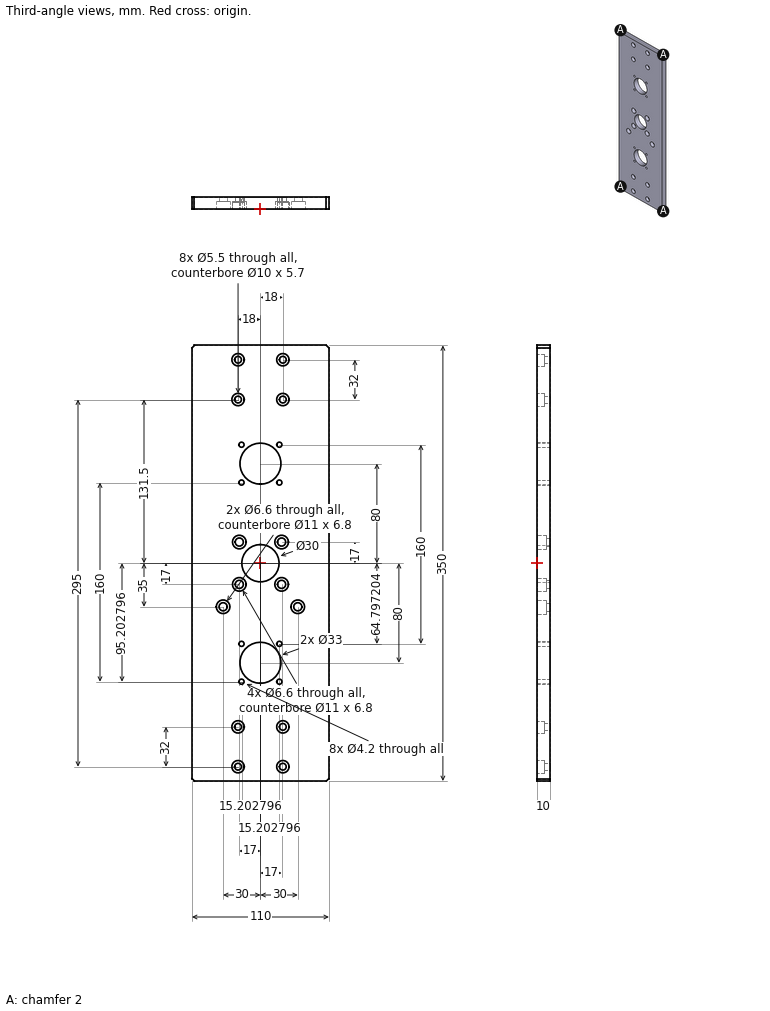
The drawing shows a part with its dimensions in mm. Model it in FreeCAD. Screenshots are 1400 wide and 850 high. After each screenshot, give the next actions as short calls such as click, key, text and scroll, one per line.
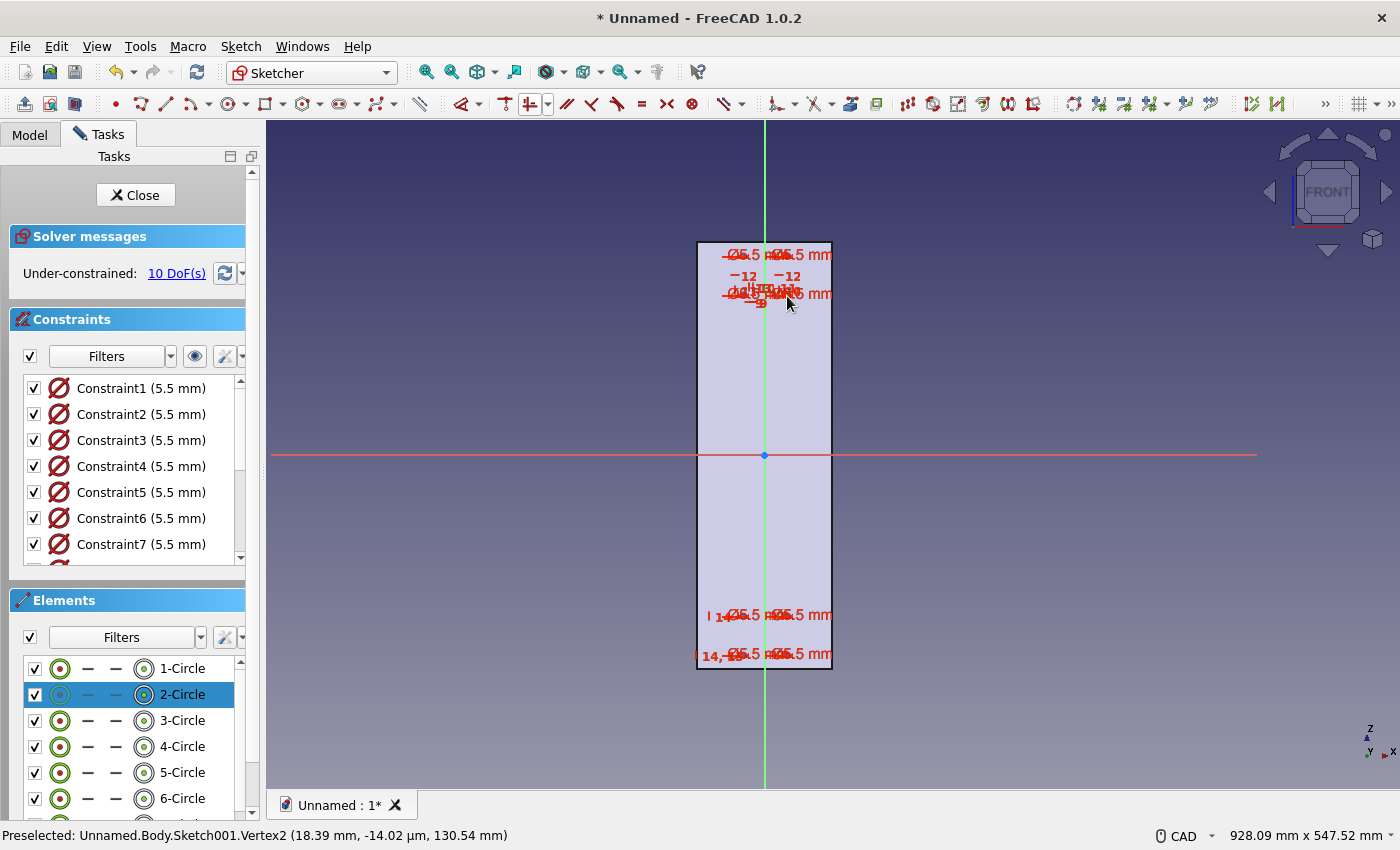
click(787, 656)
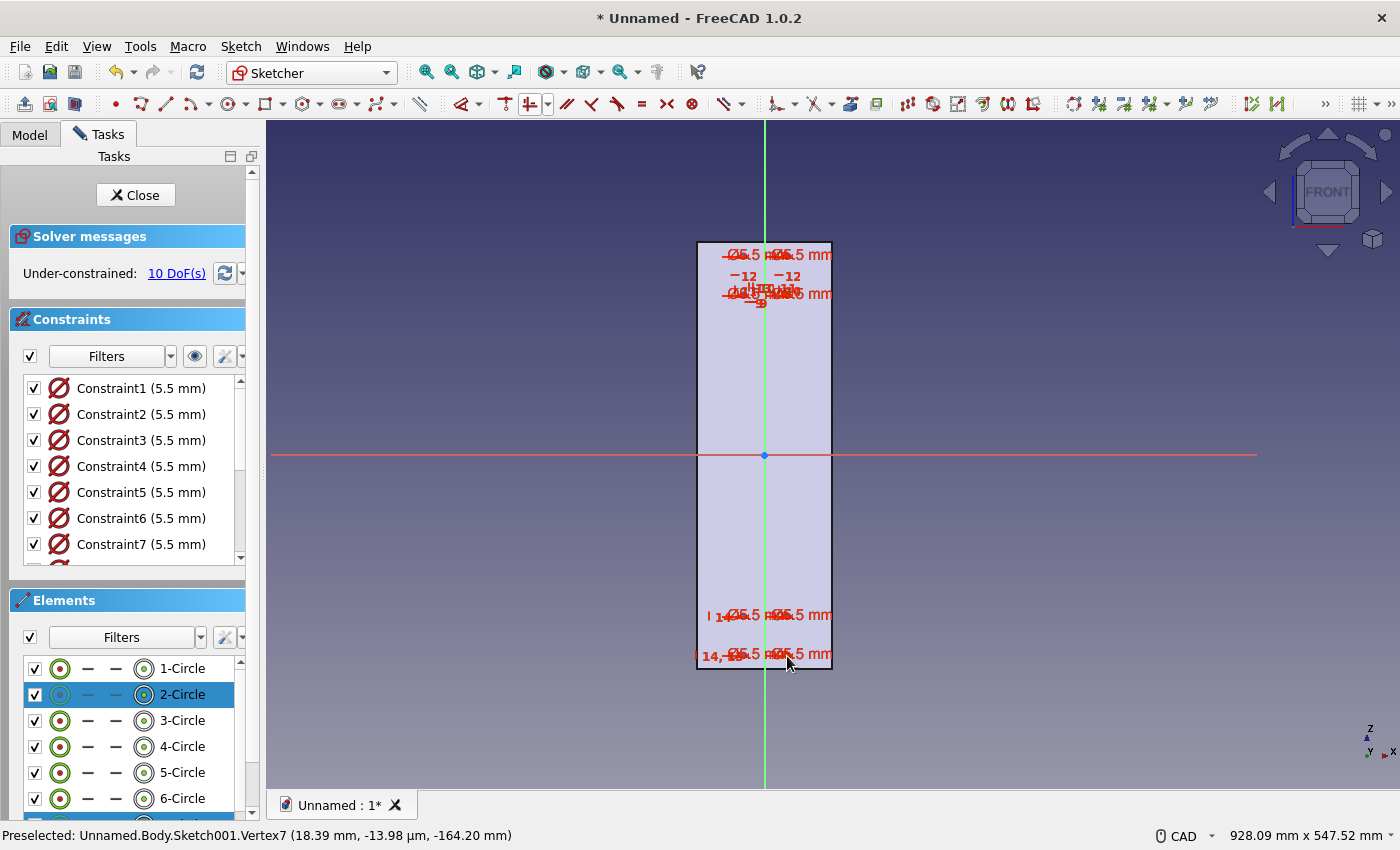
key(v)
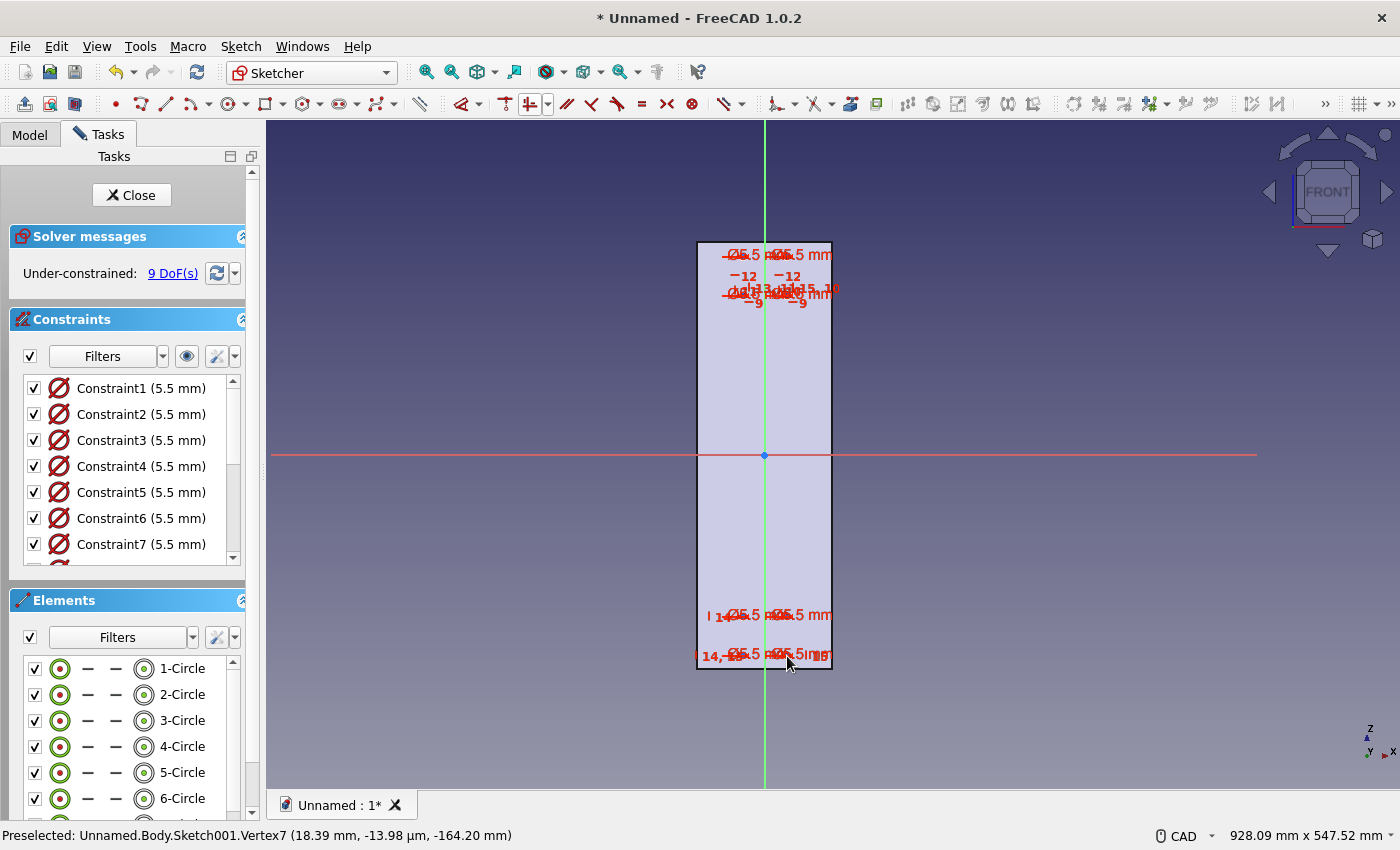
click(743, 656)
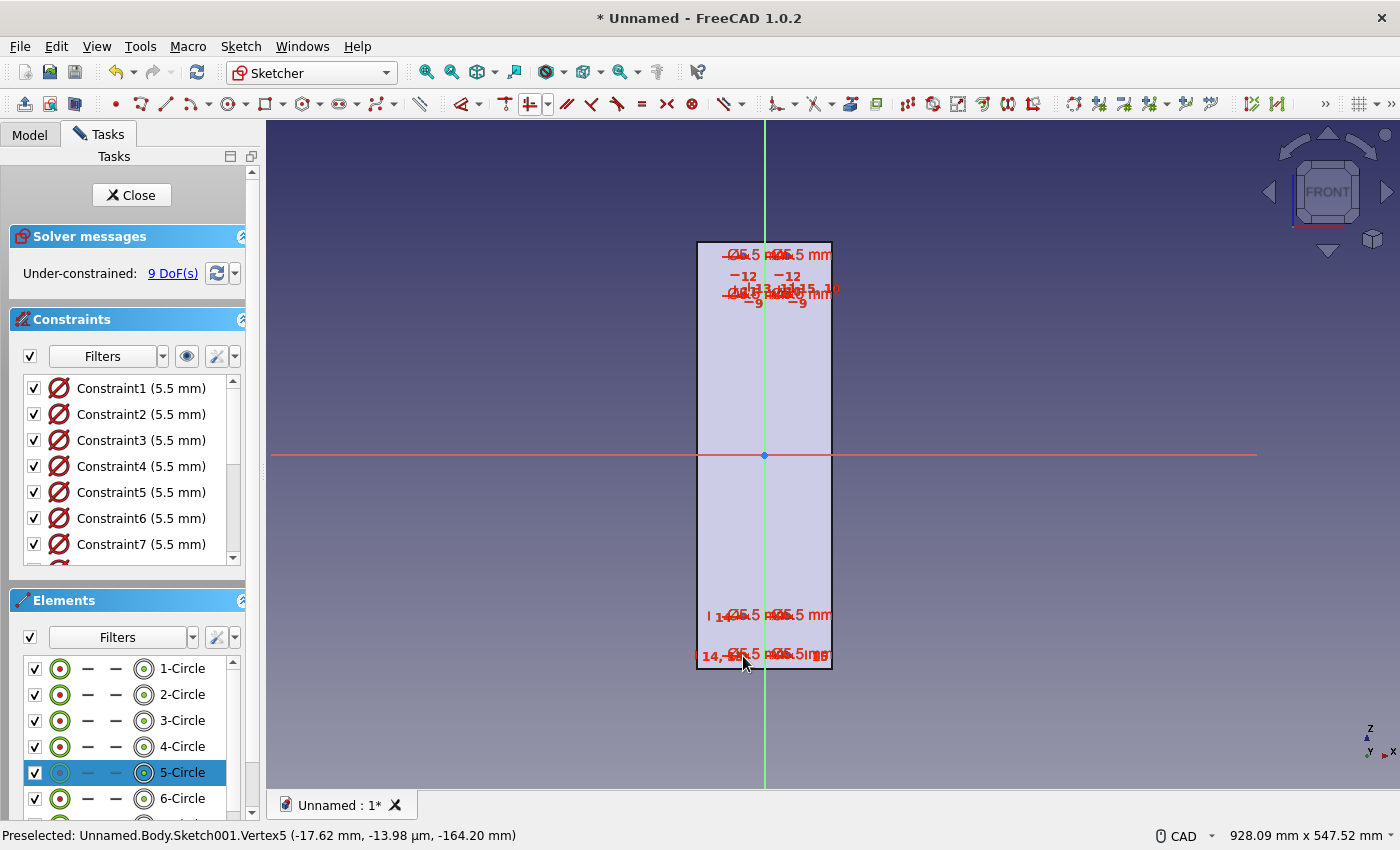
click(787, 656)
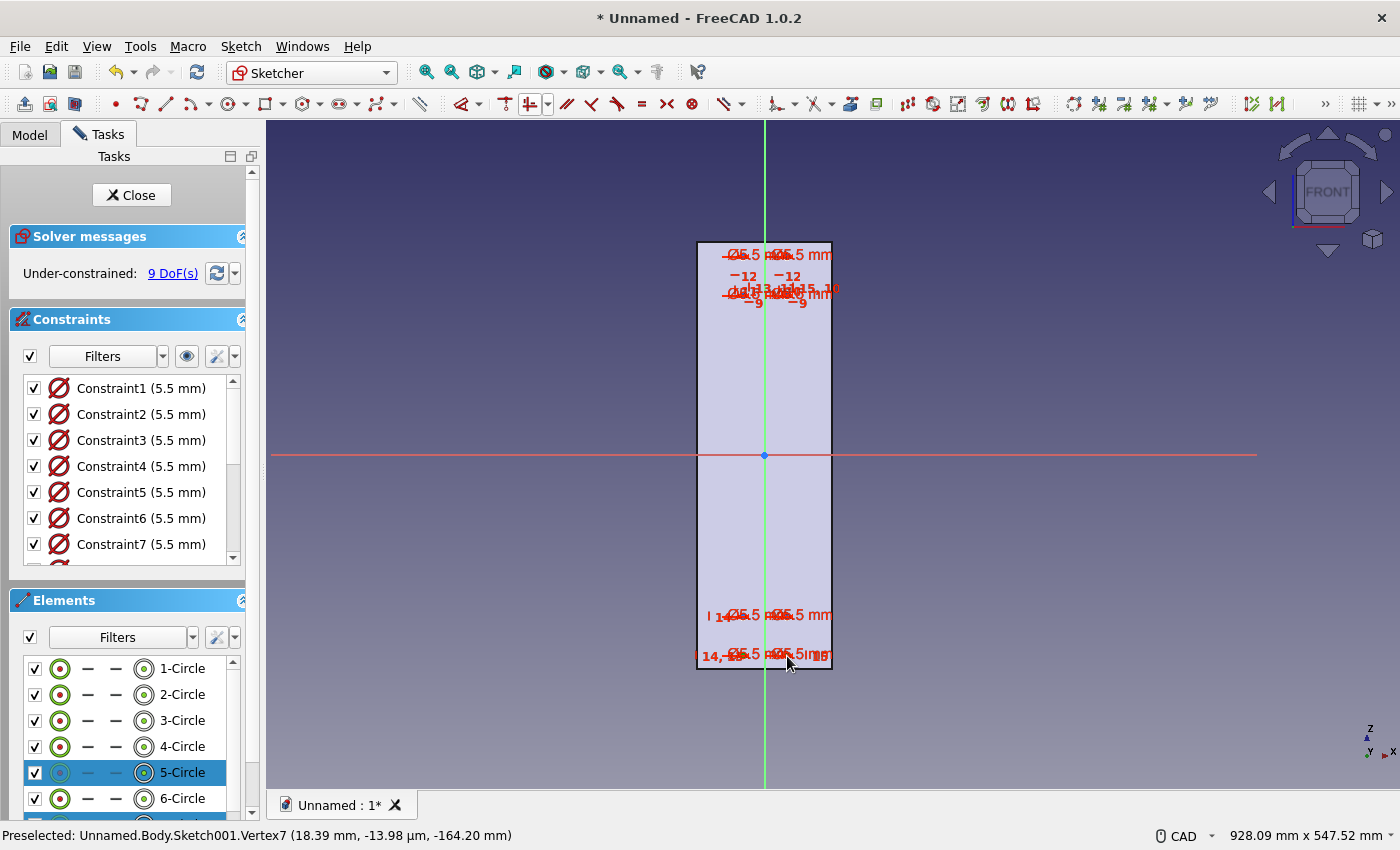
key(h)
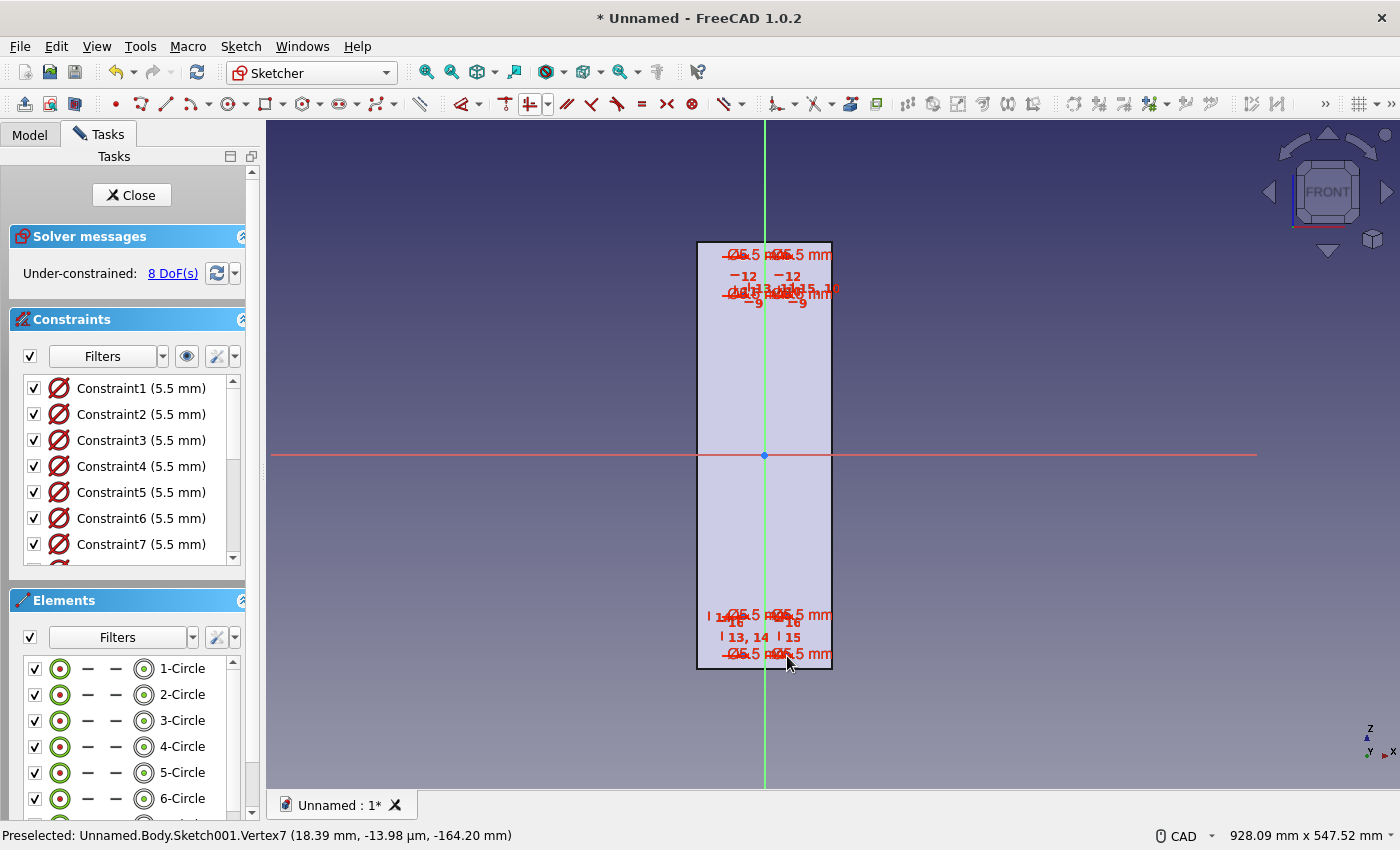
click(787, 656)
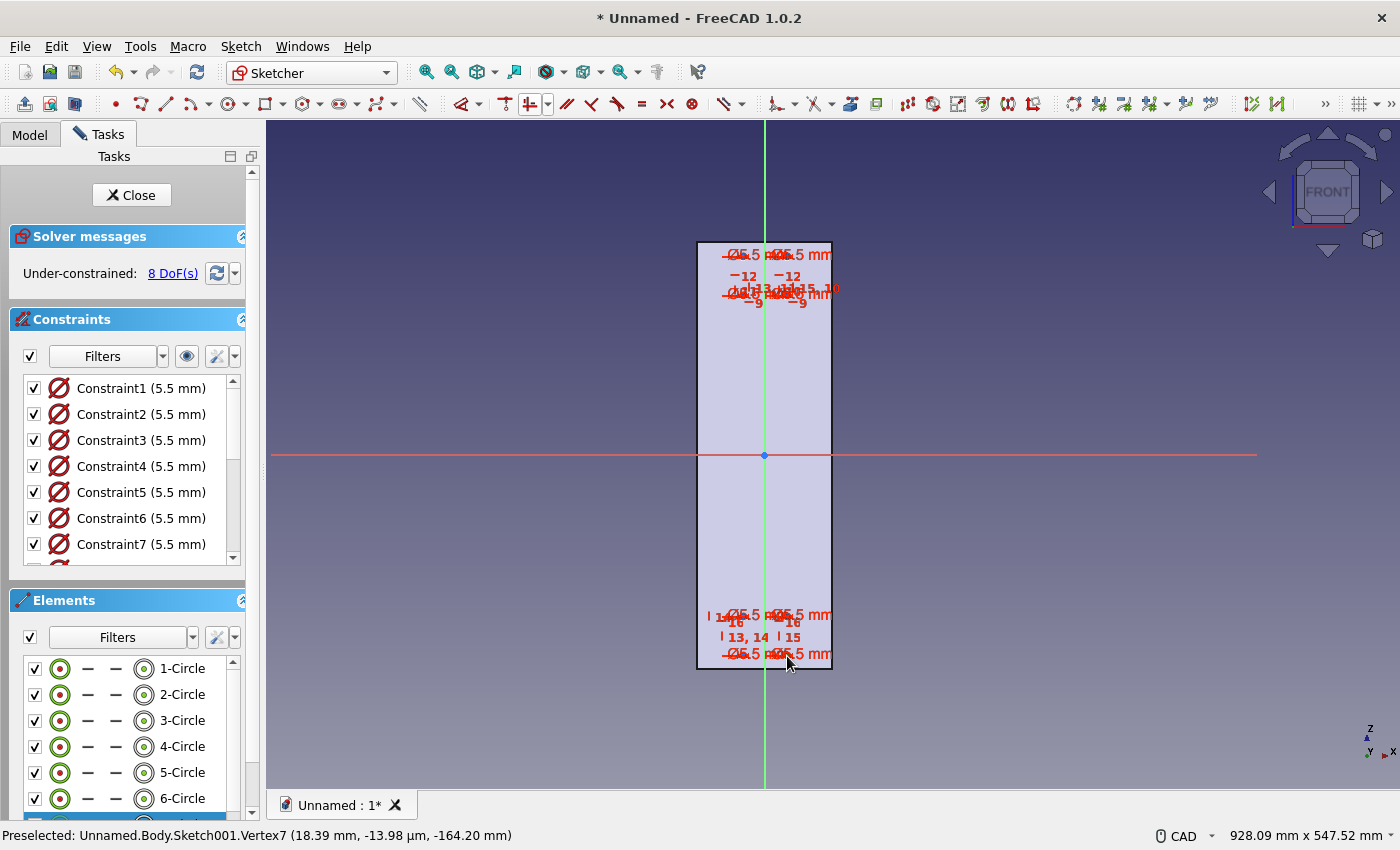
scroll(787, 617, up, 4)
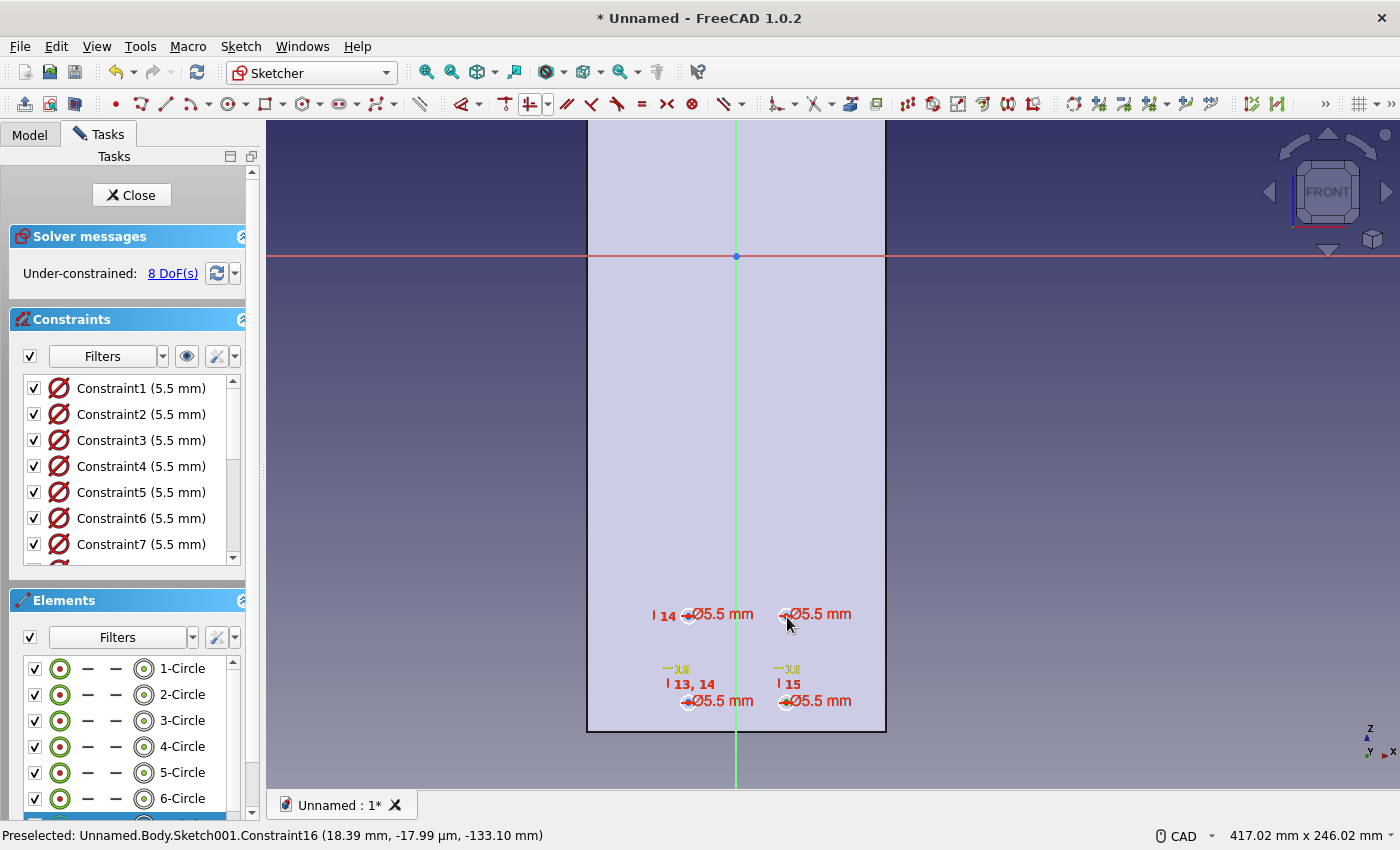
click(786, 616)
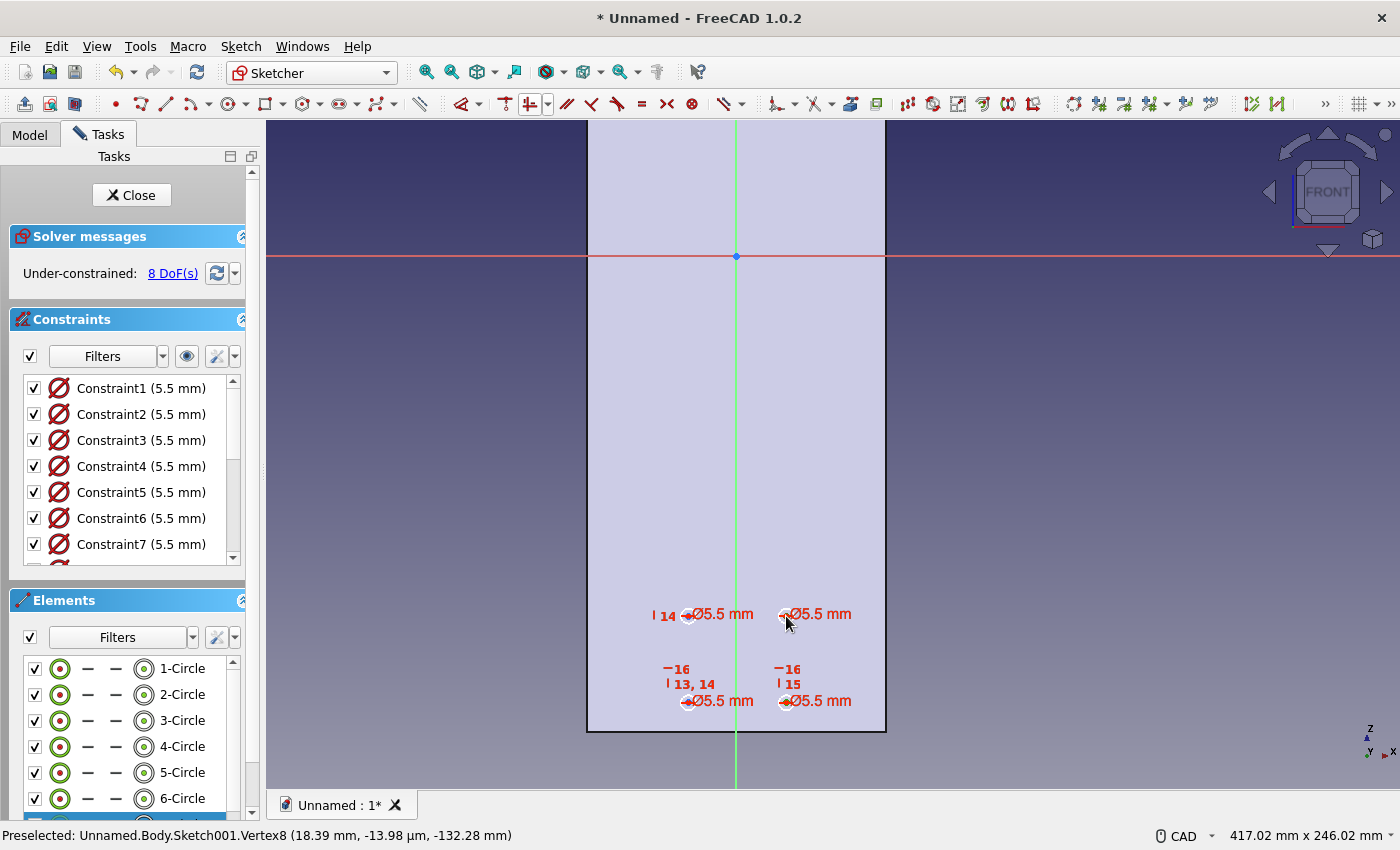
key(v)